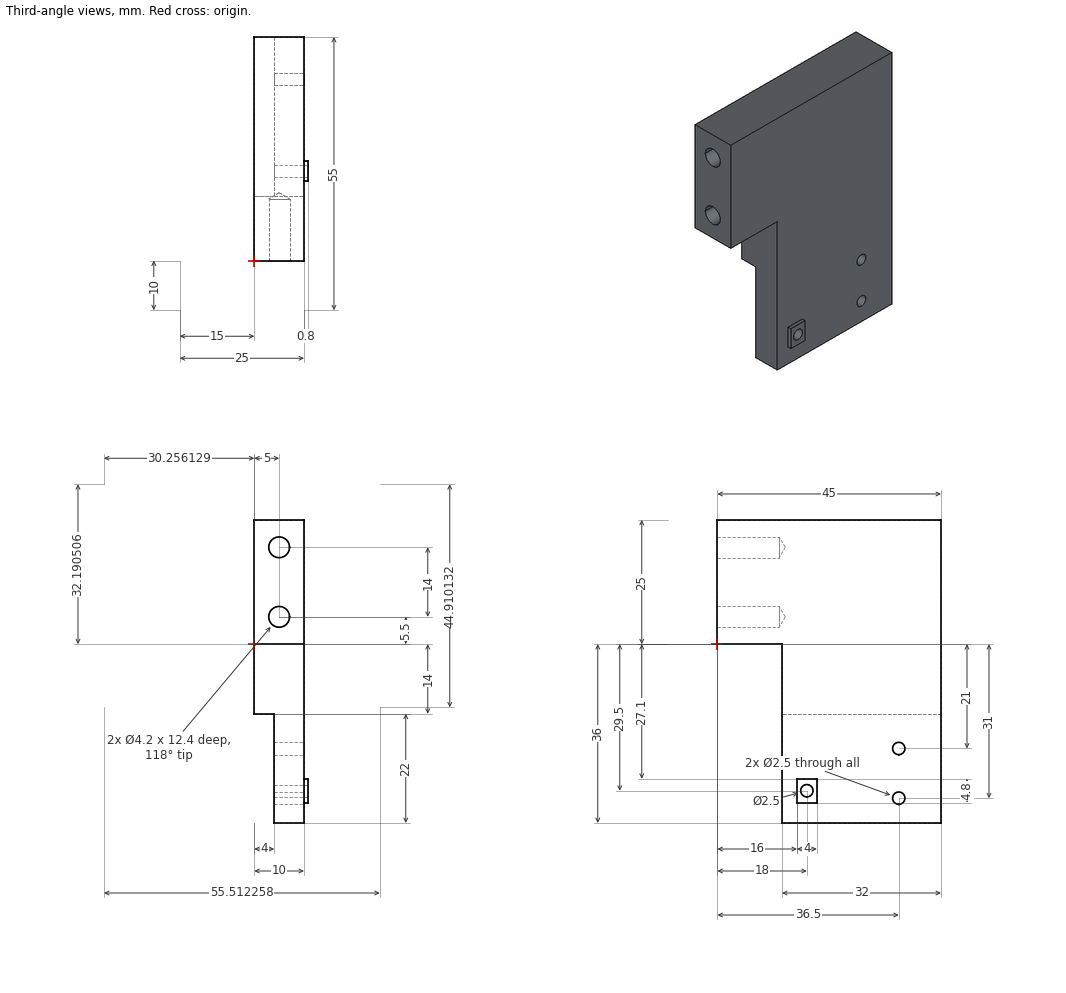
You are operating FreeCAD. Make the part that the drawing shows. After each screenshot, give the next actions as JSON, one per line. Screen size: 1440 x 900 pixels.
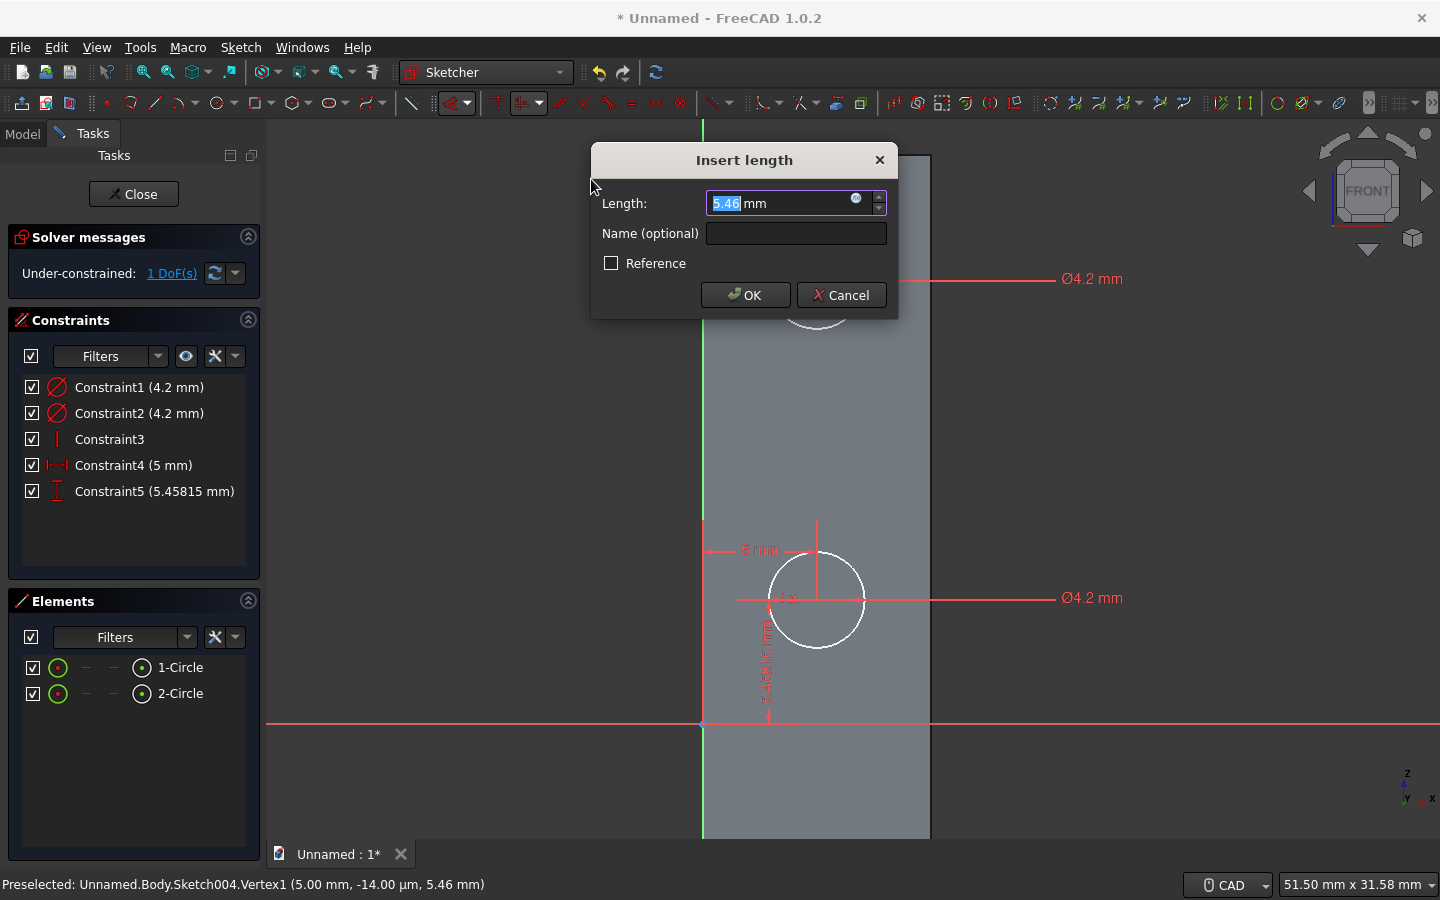
{"action": "type", "text": "5.5"}
{"action": "key", "text": "Return"}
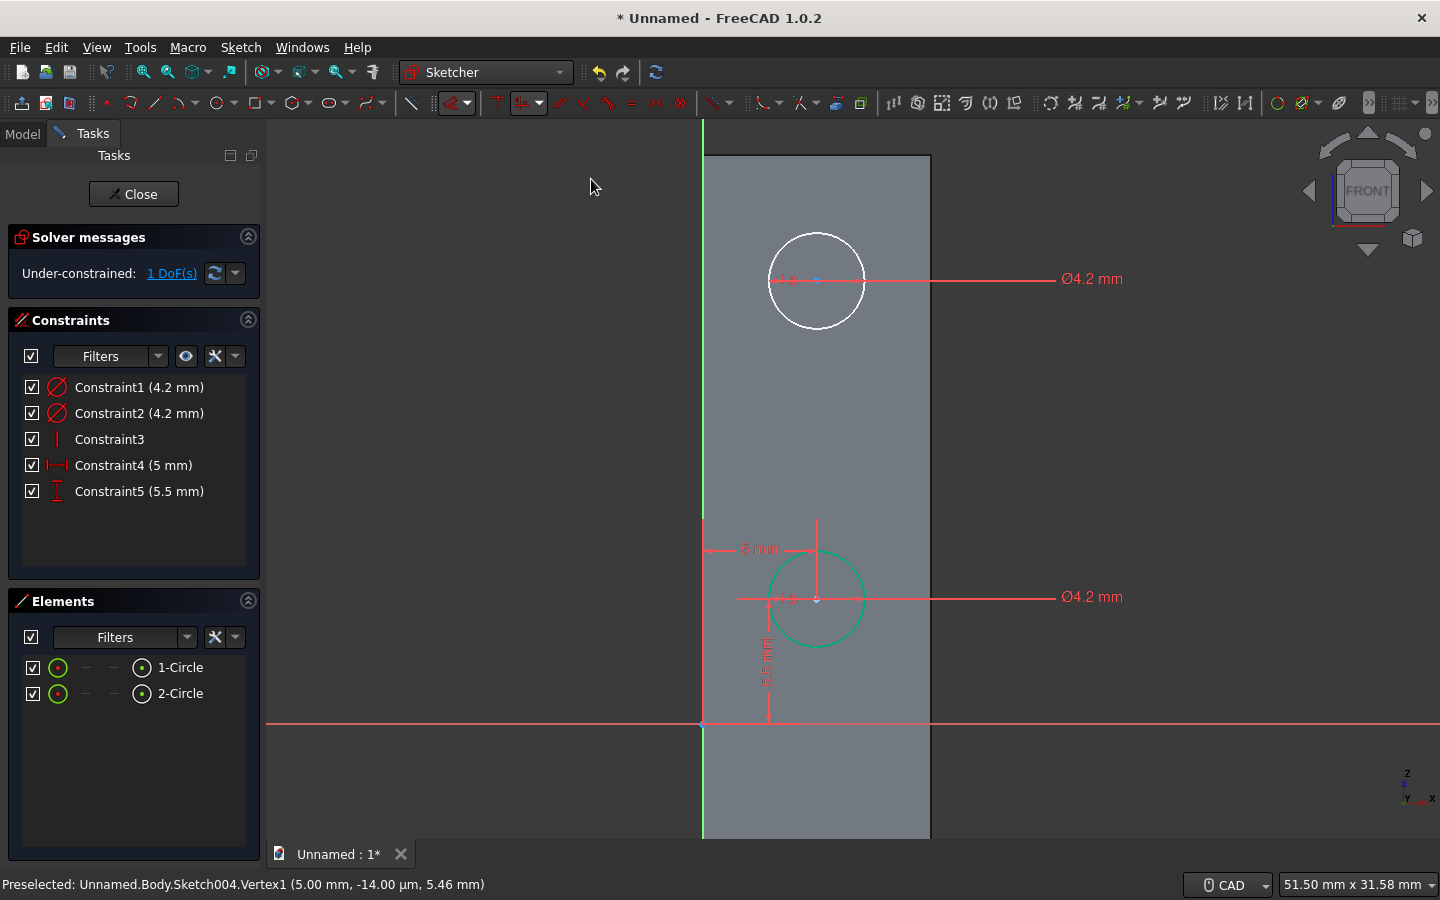
{"action": "left_click", "coordinate": [817, 599]}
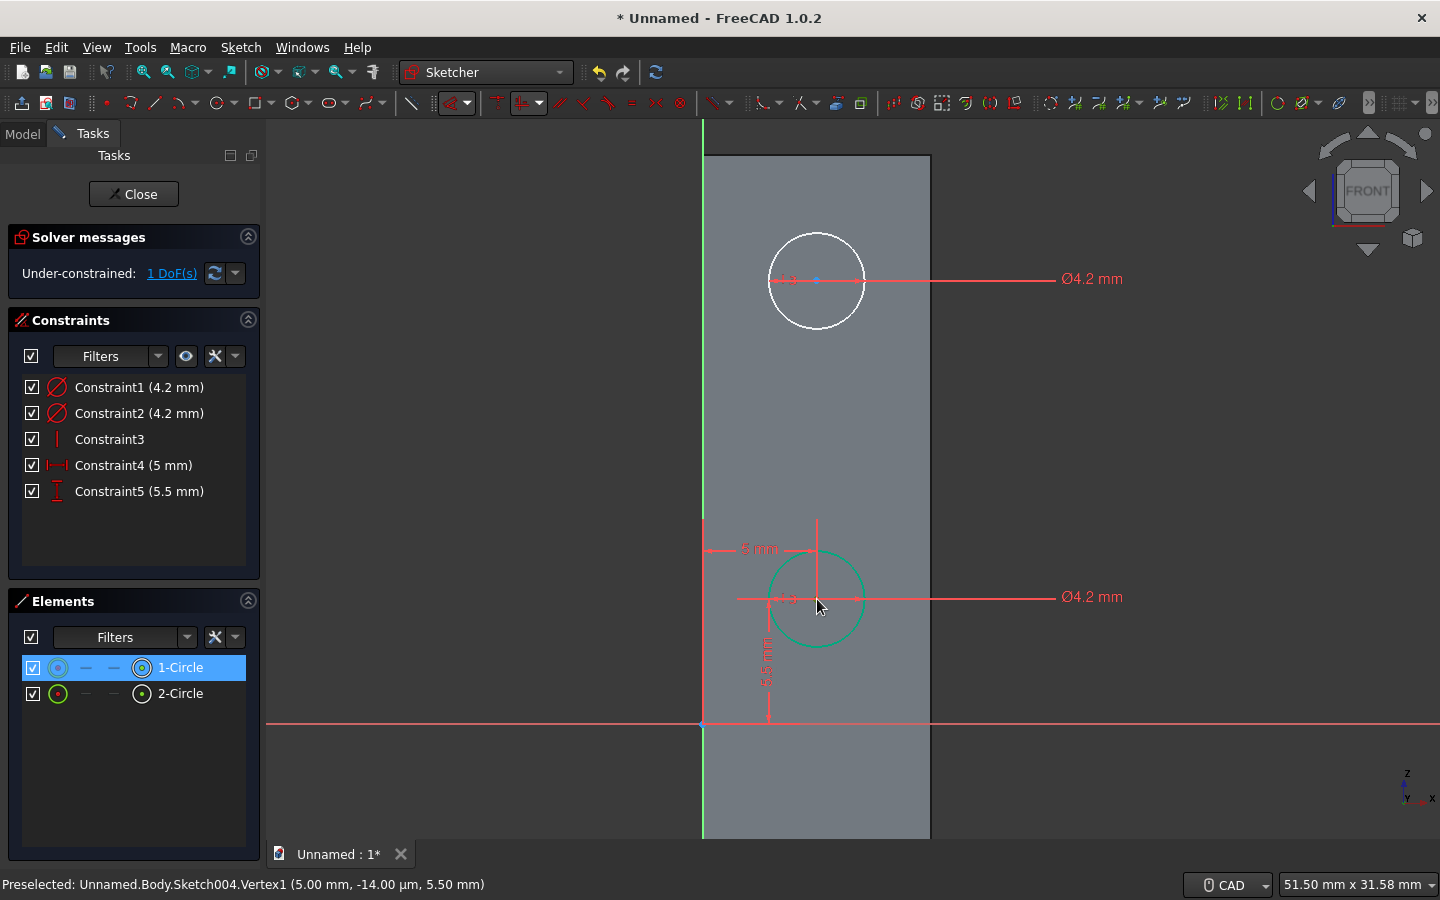
{"action": "left_click", "coordinate": [817, 281]}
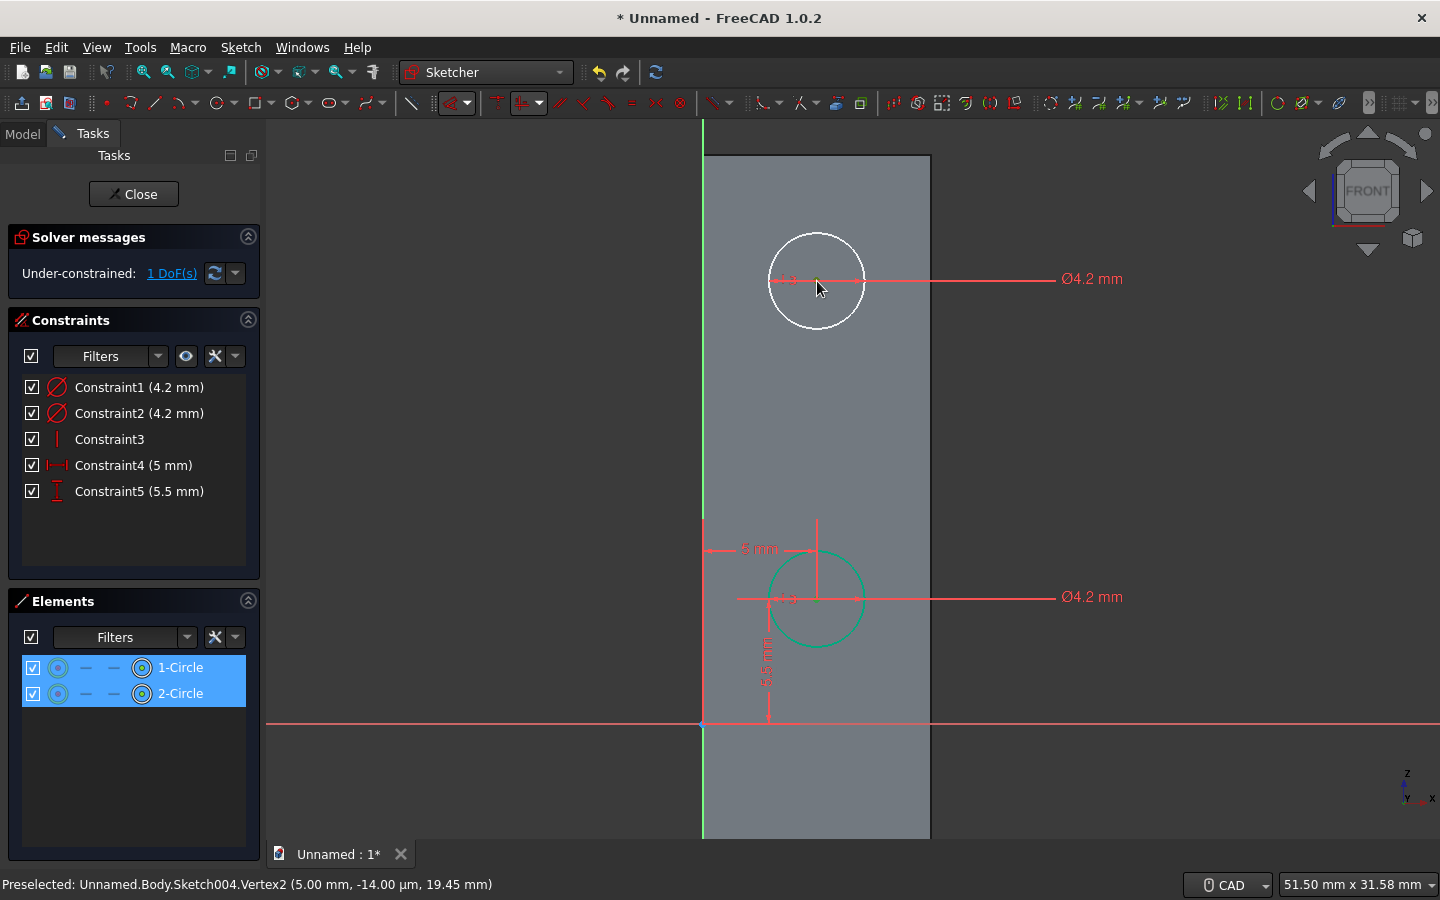
{"action": "key", "text": "i"}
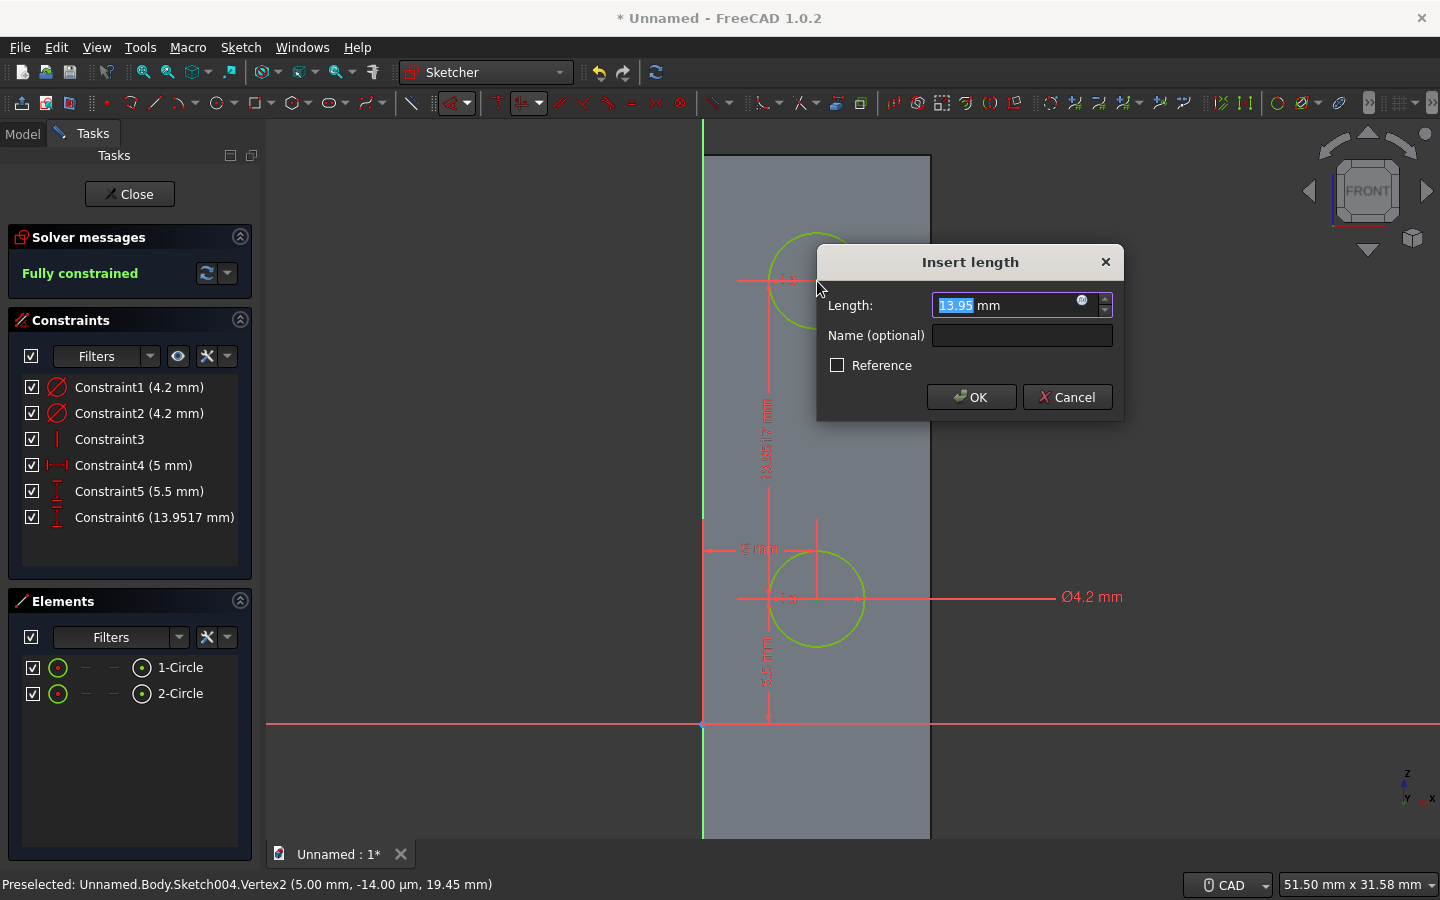
{"action": "type", "text": "14"}
{"action": "key", "text": "Return"}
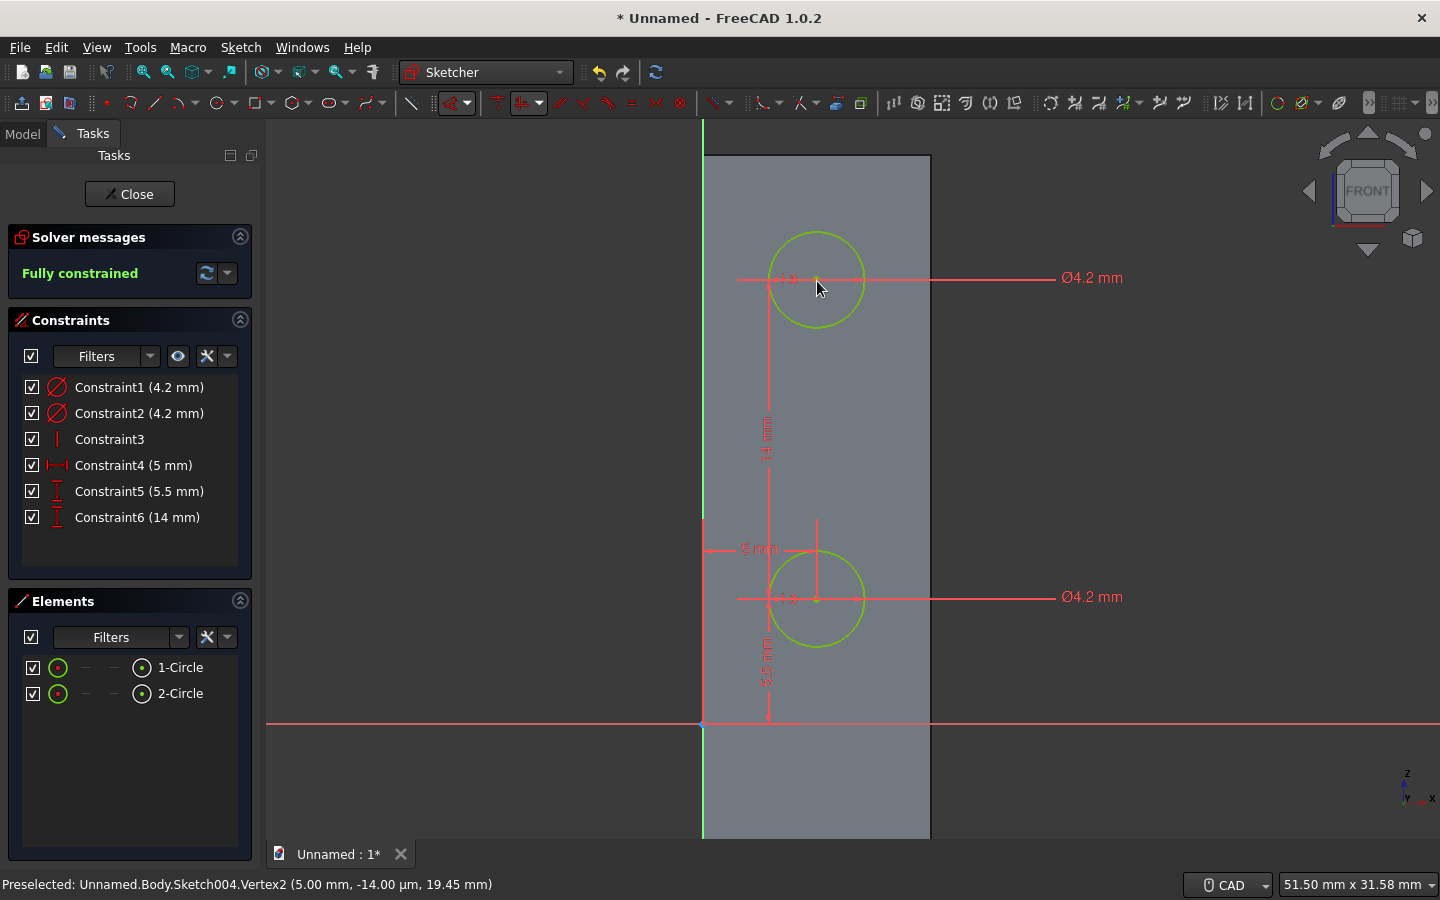
{"action": "left_click", "coordinate": [130, 194]}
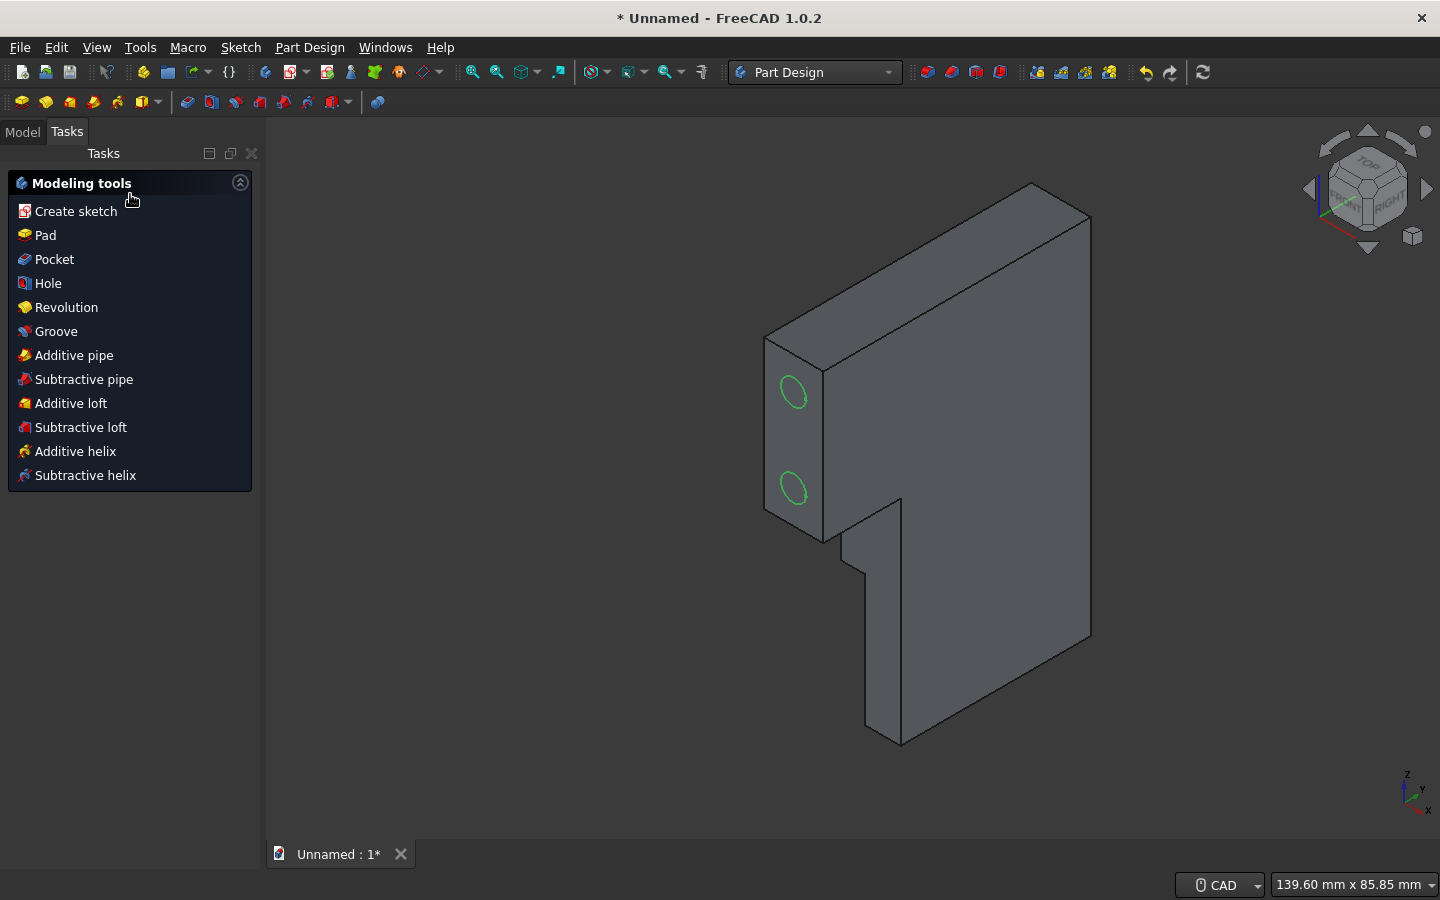
{"action": "left_click", "coordinate": [212, 102]}